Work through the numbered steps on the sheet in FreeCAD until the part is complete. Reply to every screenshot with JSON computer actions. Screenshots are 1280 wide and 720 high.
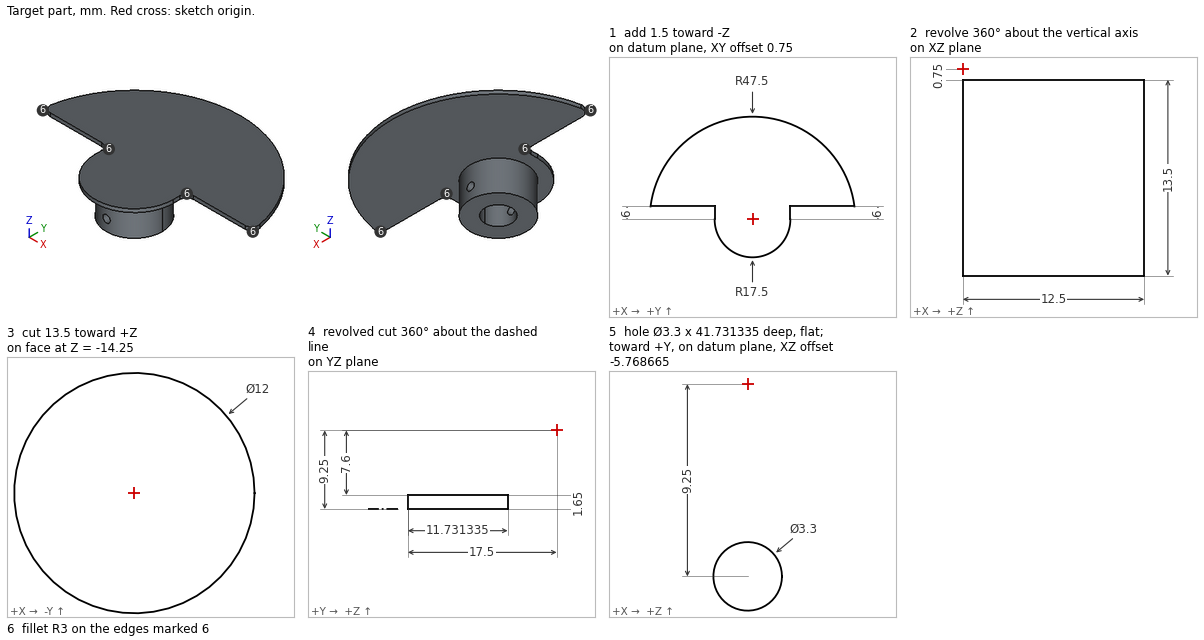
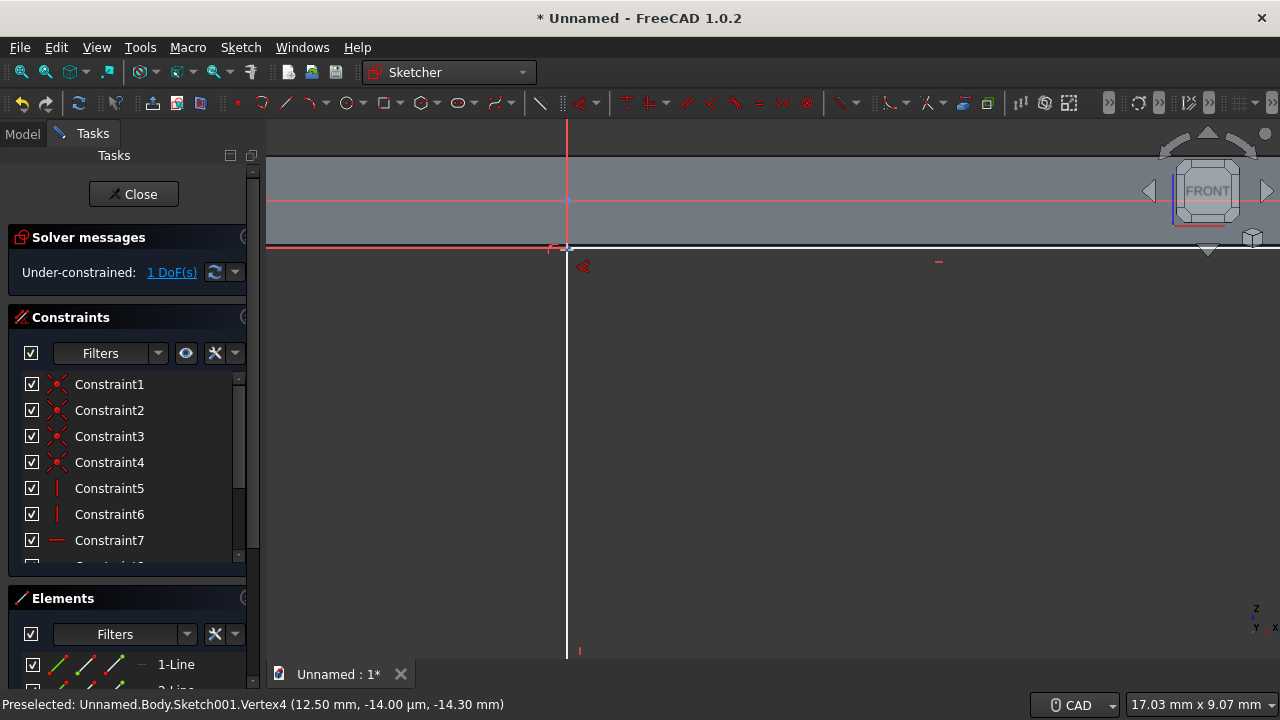
{"action": "left_click", "coordinate": [567, 248]}
{"action": "left_click", "coordinate": [533, 224]}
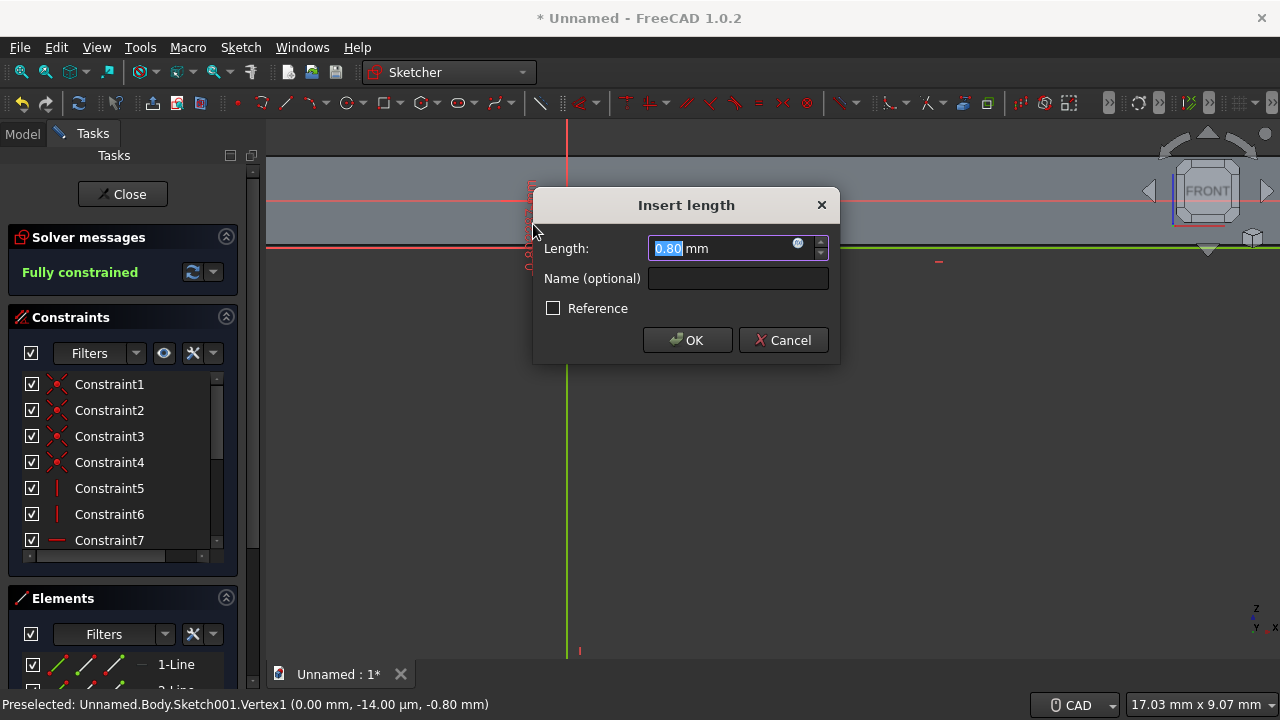
{"action": "type", "text": "0.75"}
{"action": "key", "text": "Return"}
{"action": "key", "text": "Escape"}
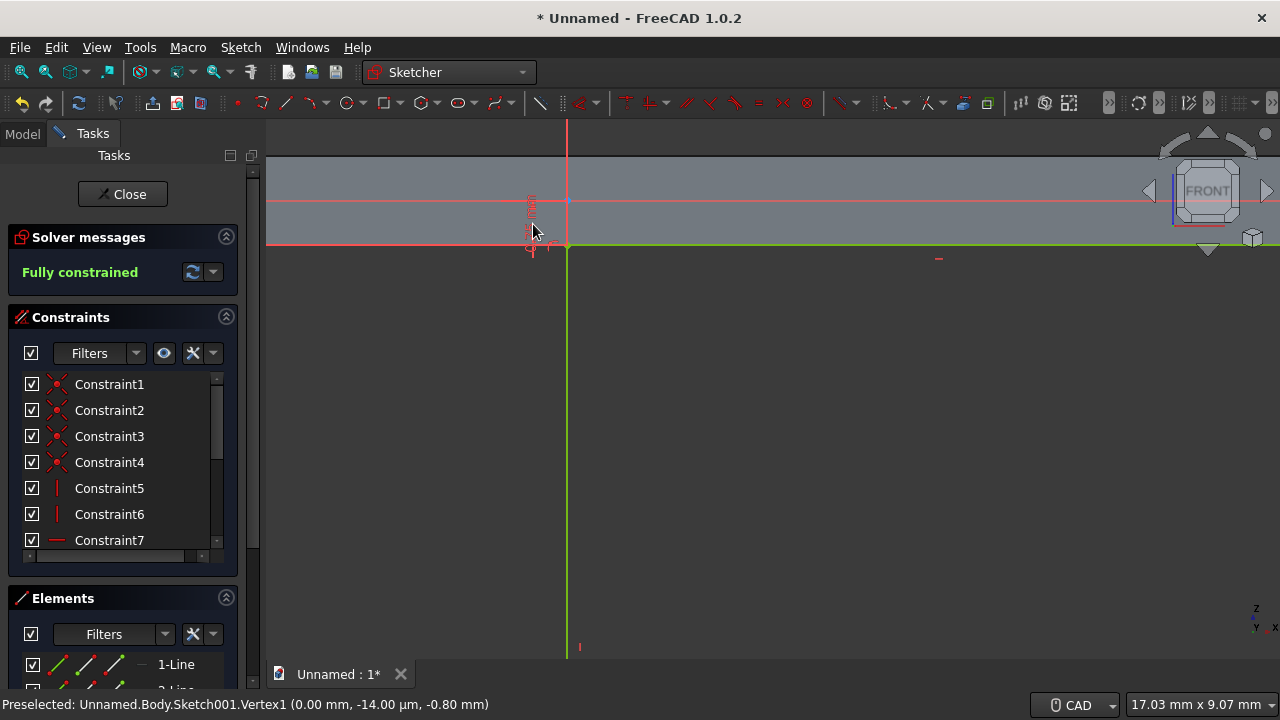
{"action": "left_click", "coordinate": [123, 194]}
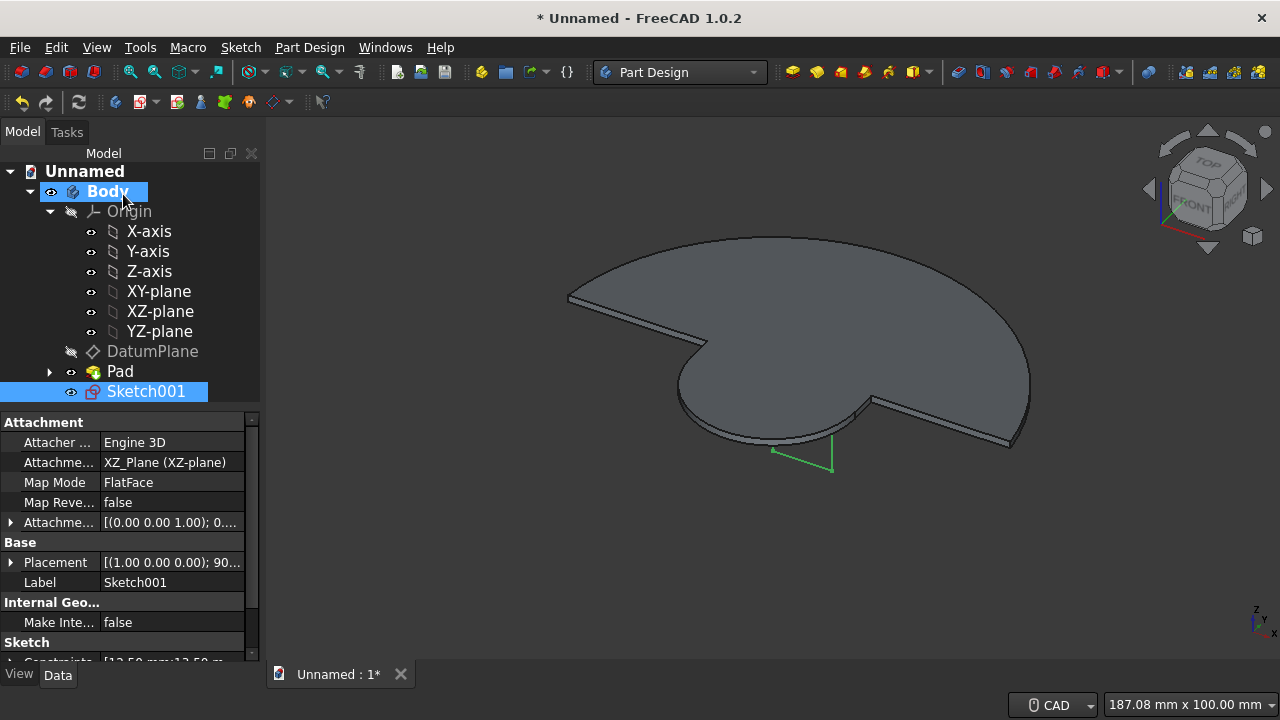
{"action": "left_click", "coordinate": [818, 72]}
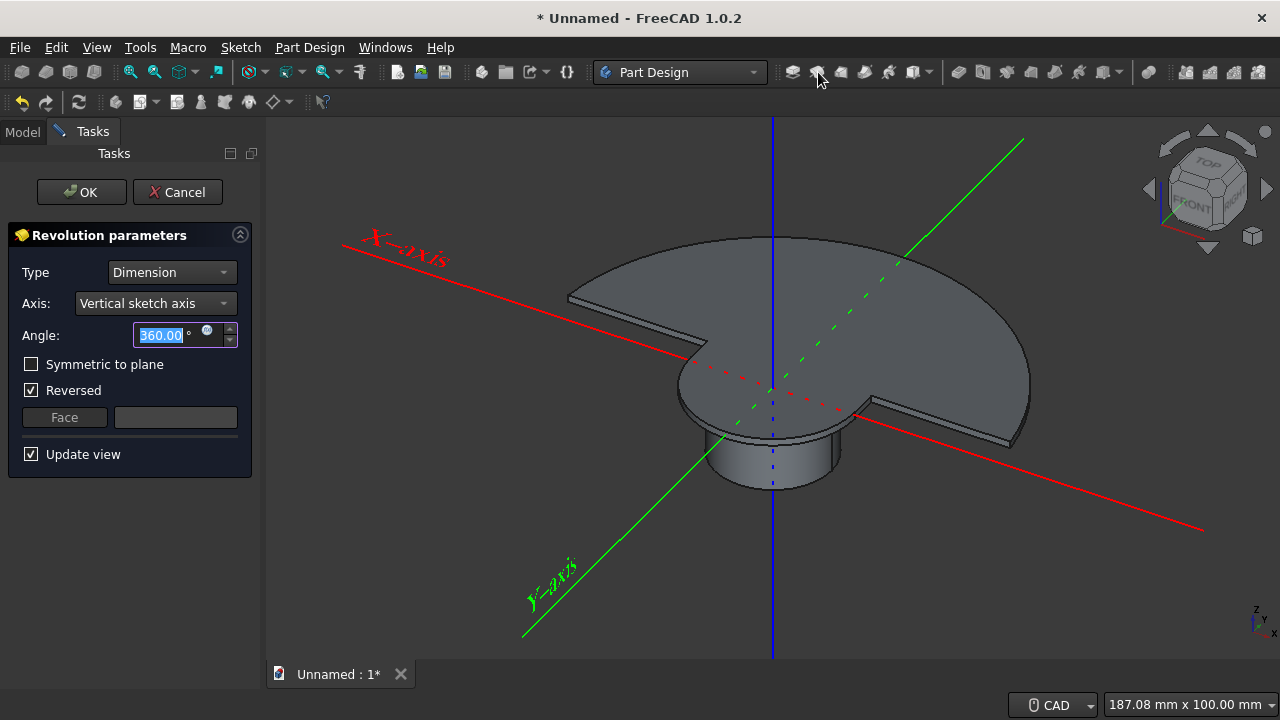
{"action": "left_click", "coordinate": [82, 192]}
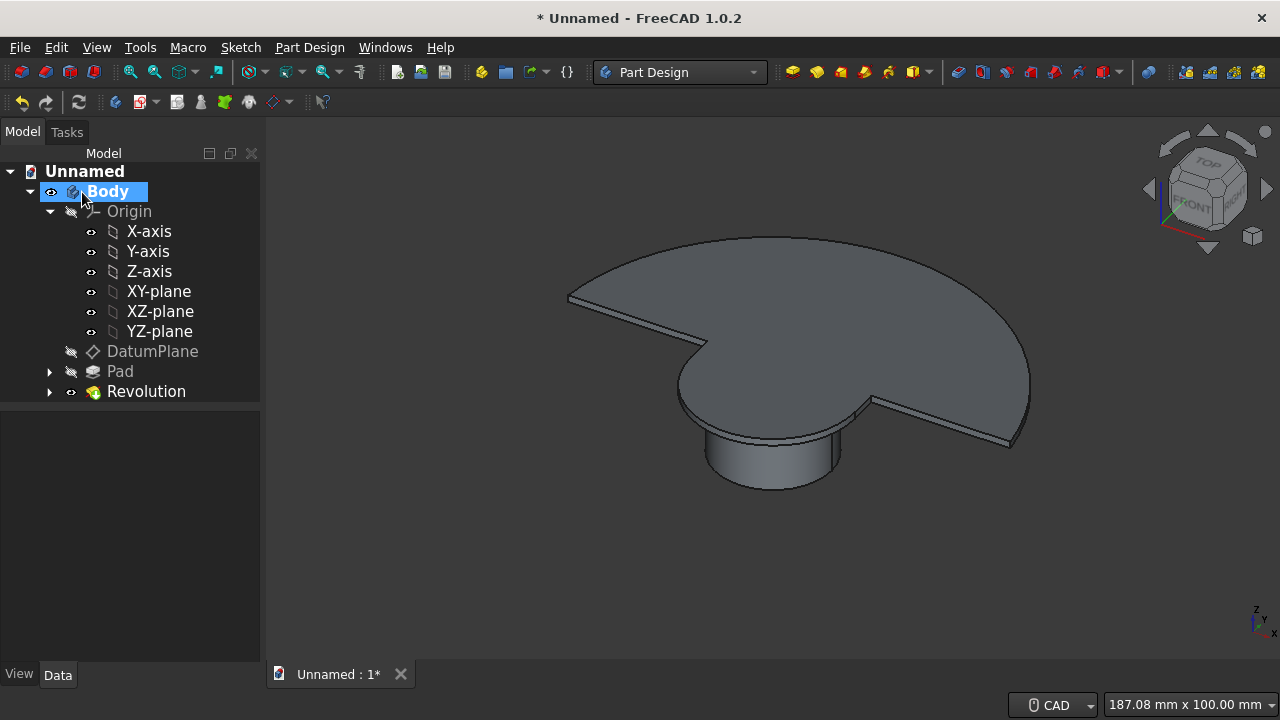
{"action": "key", "text": "5"}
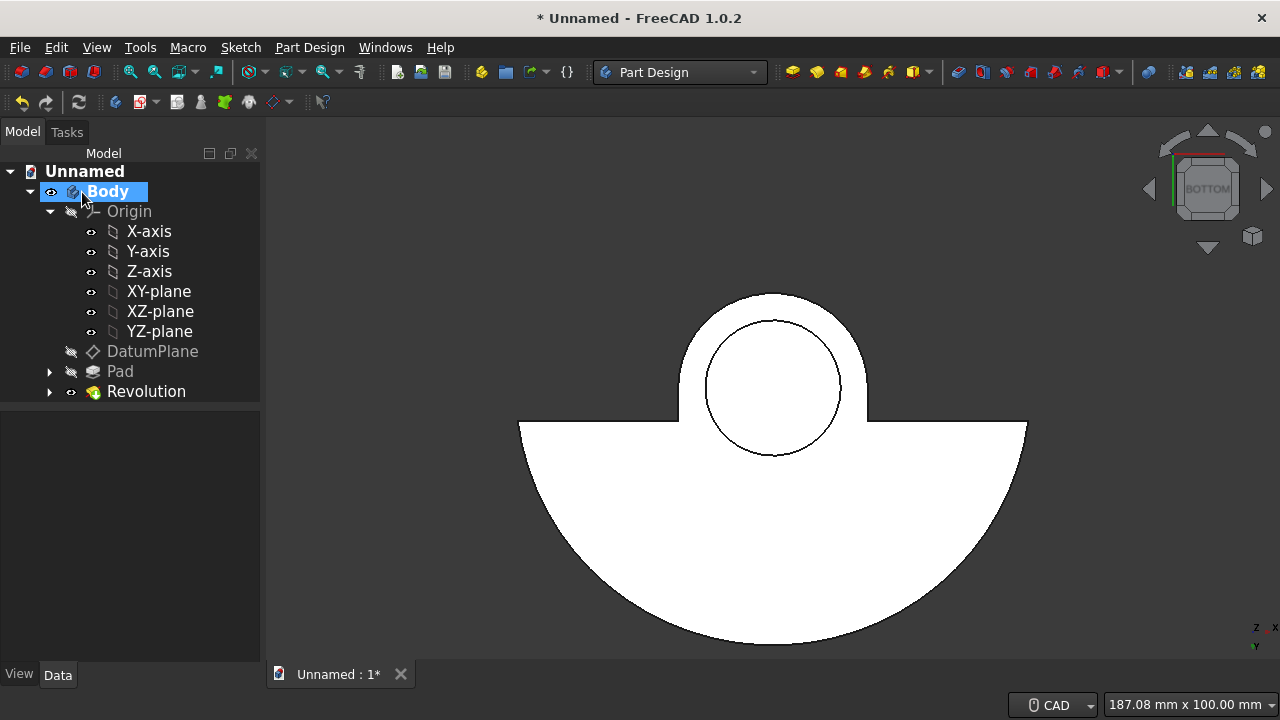
{"action": "left_click", "coordinate": [773, 387]}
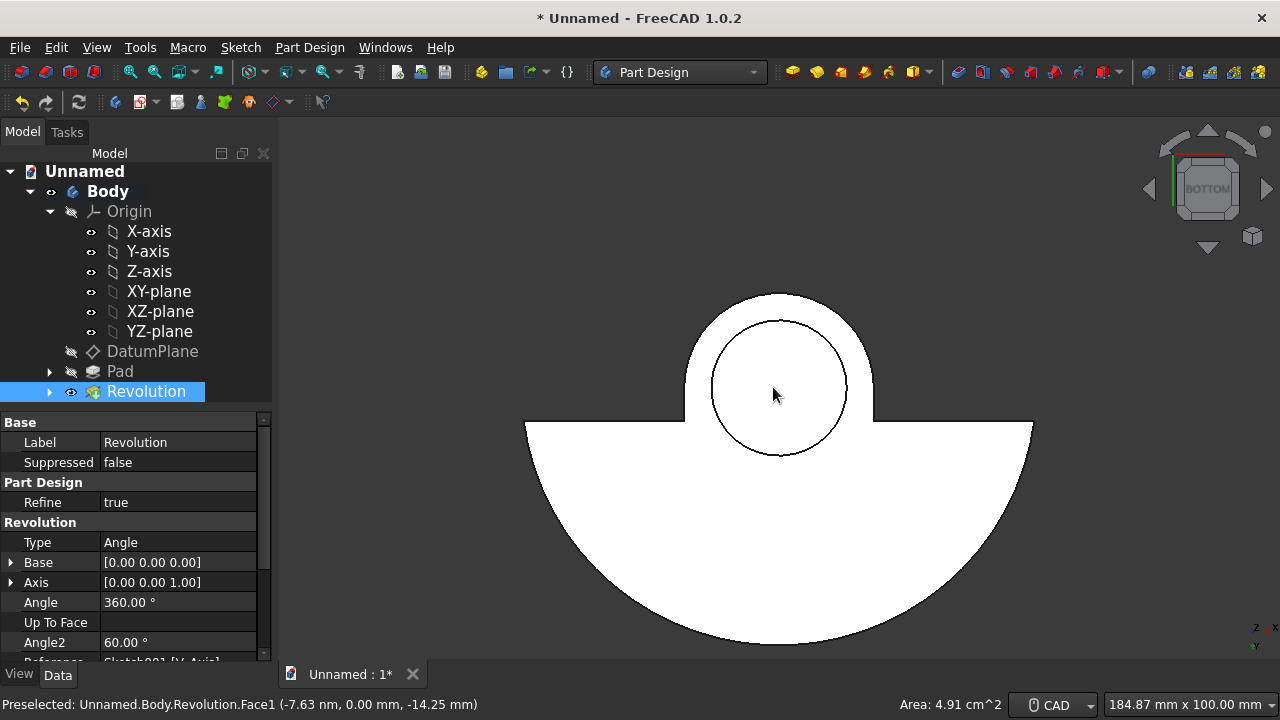
{"action": "left_click", "coordinate": [140, 102]}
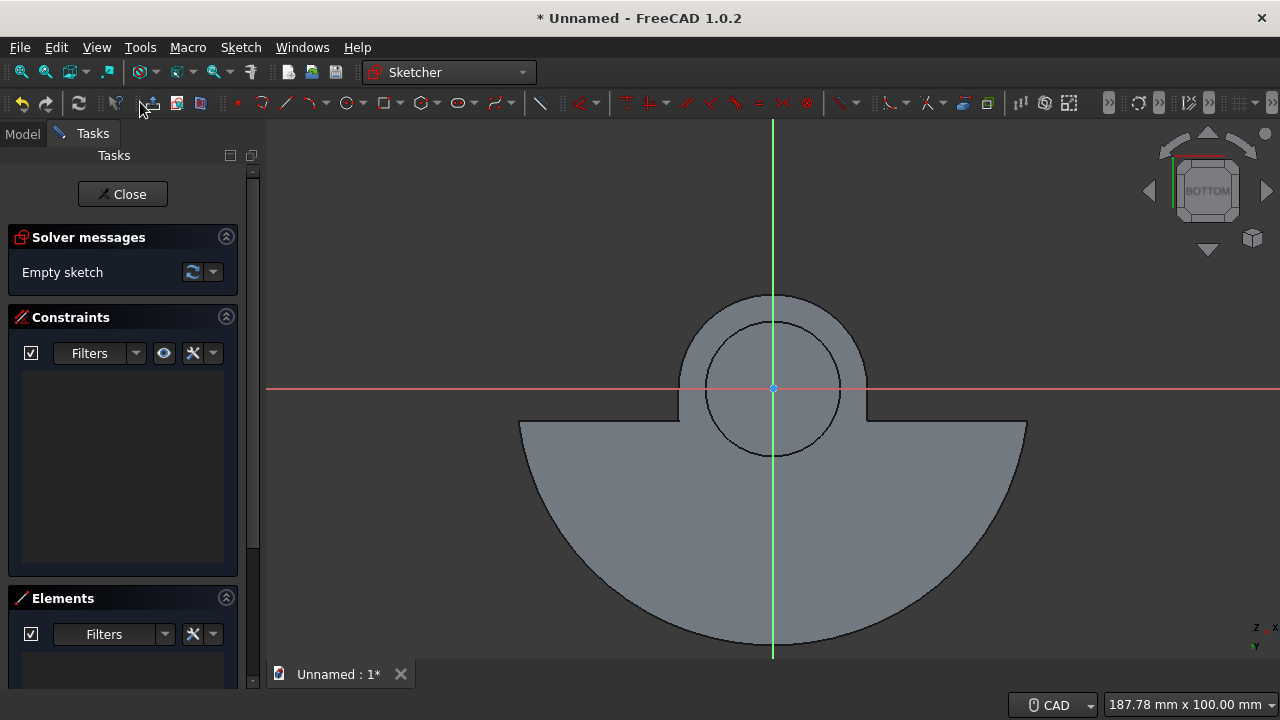
{"action": "scroll", "coordinate": [790, 389], "scroll_direction": "up", "scroll_amount": 8}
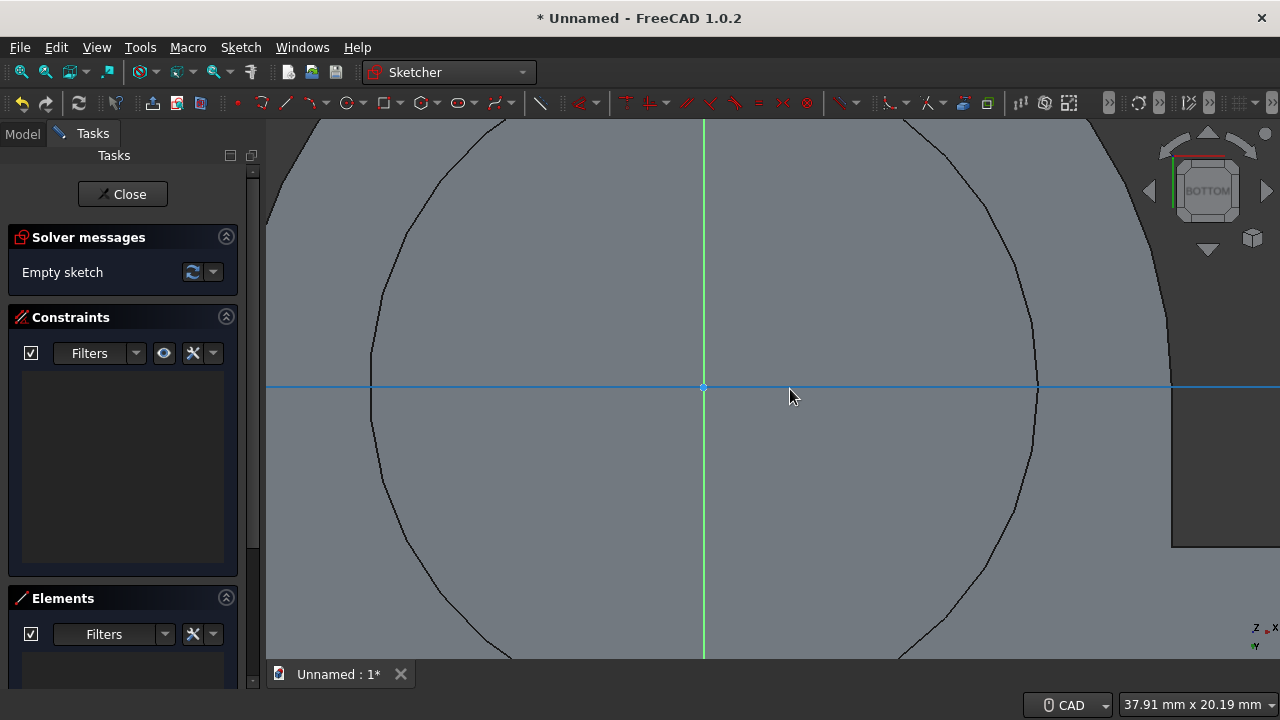
{"action": "key", "text": "g c"}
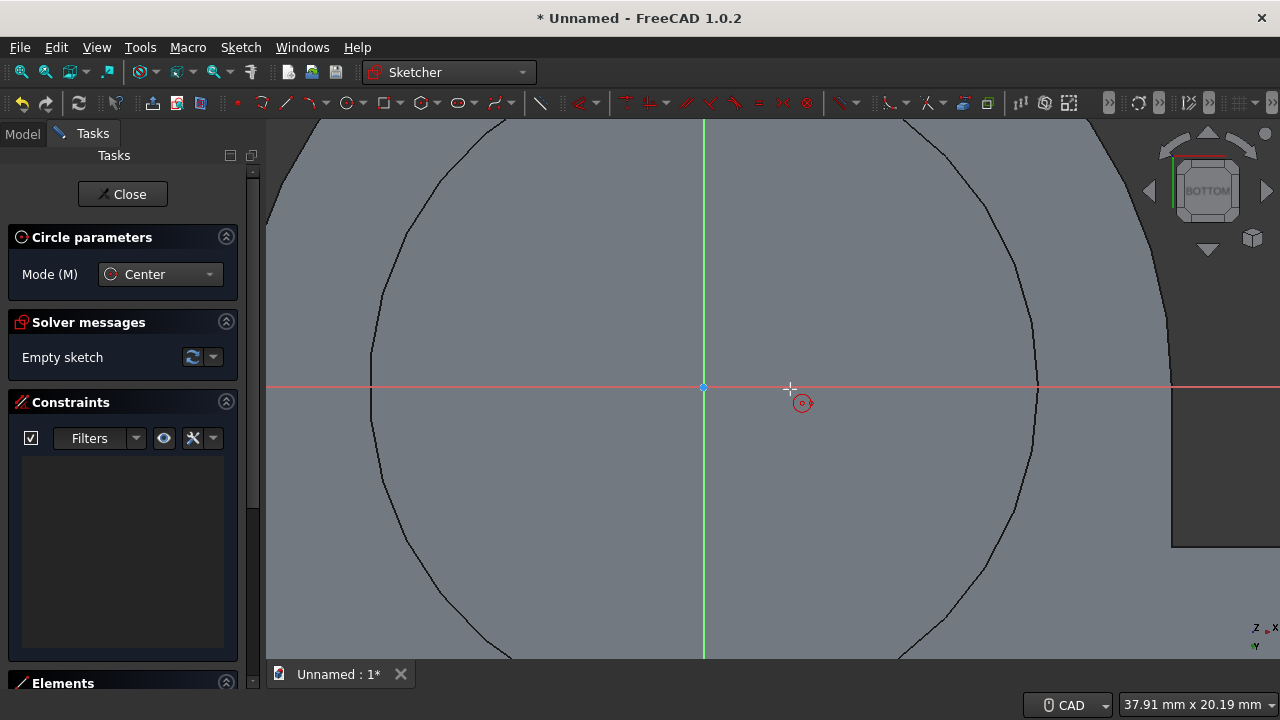
{"action": "left_click", "coordinate": [704, 387]}
{"action": "mouse_move", "coordinate": [817, 274]}